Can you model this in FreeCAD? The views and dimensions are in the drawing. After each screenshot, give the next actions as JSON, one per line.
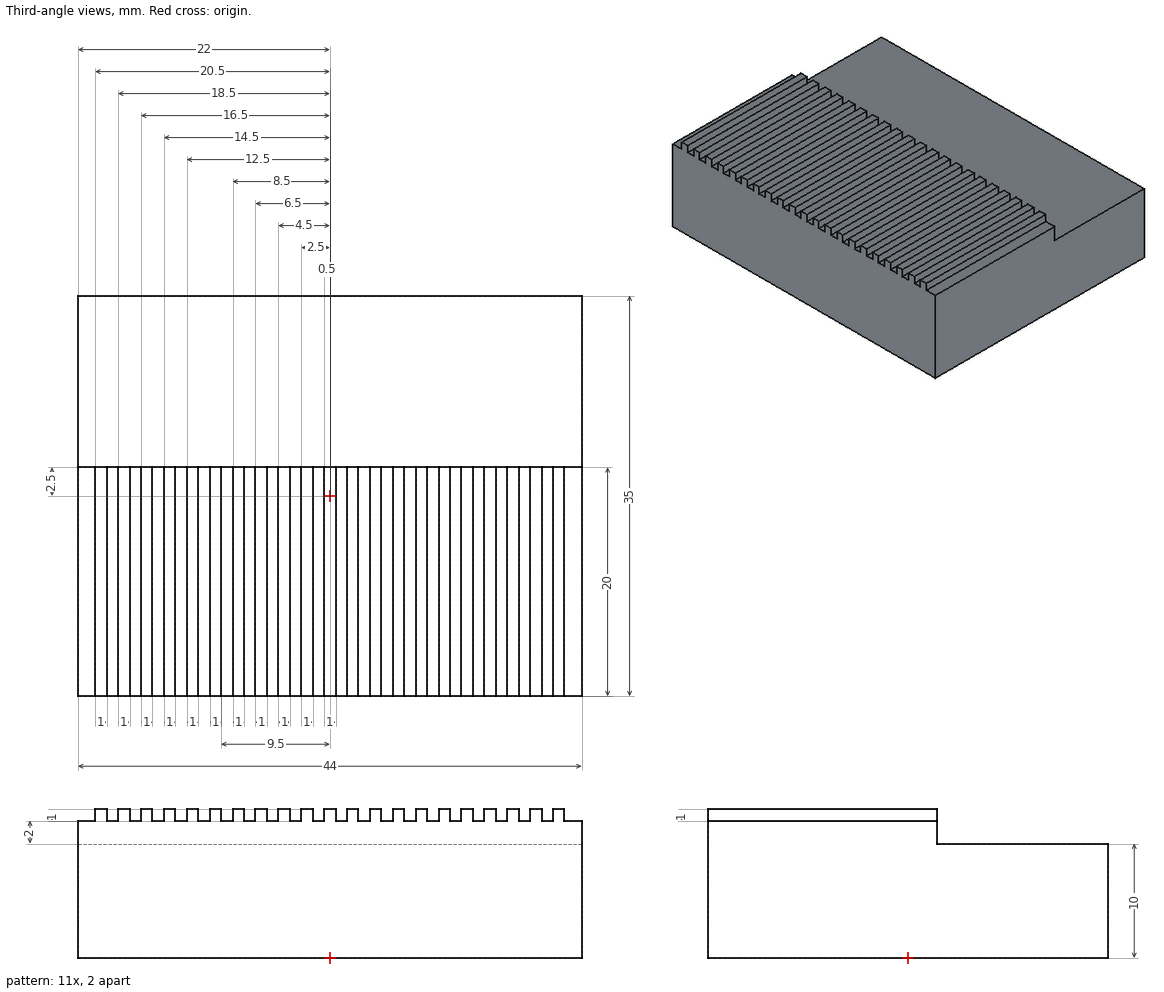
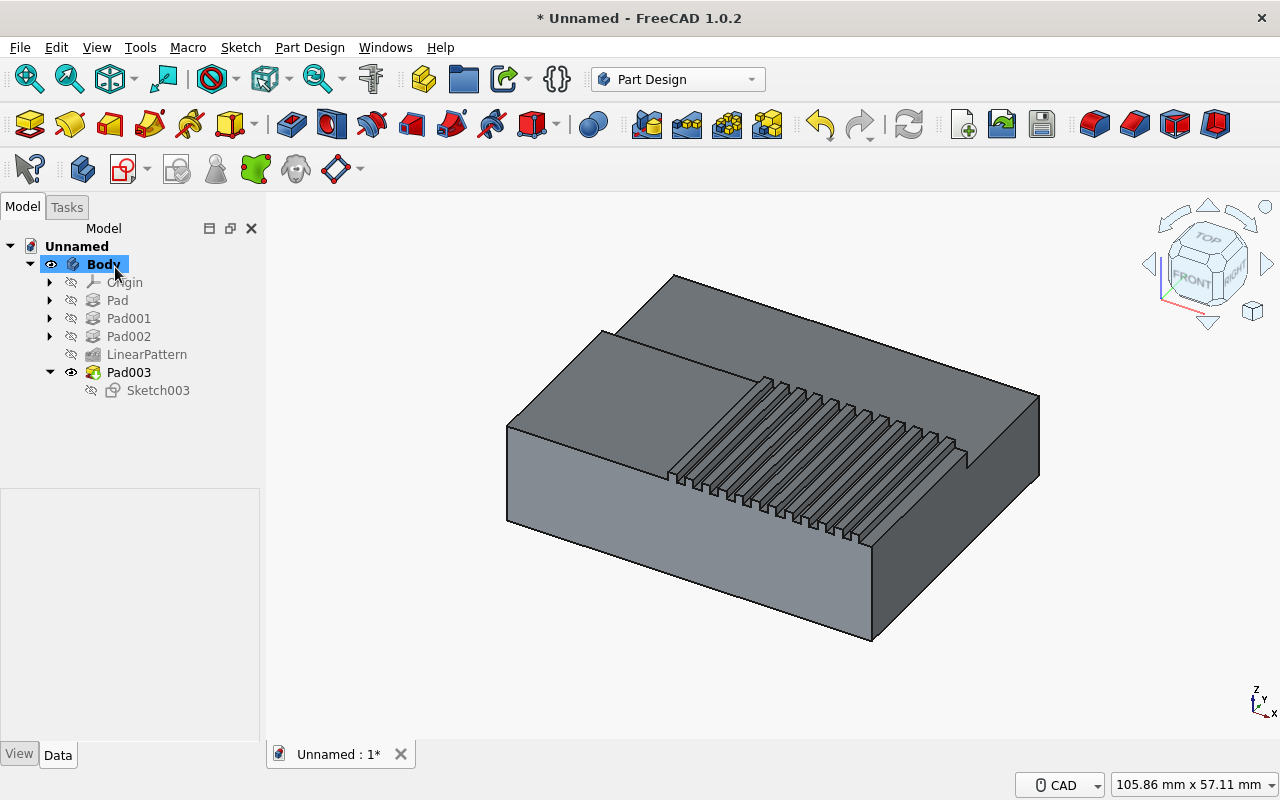
{"action": "left_click", "coordinate": [635, 404]}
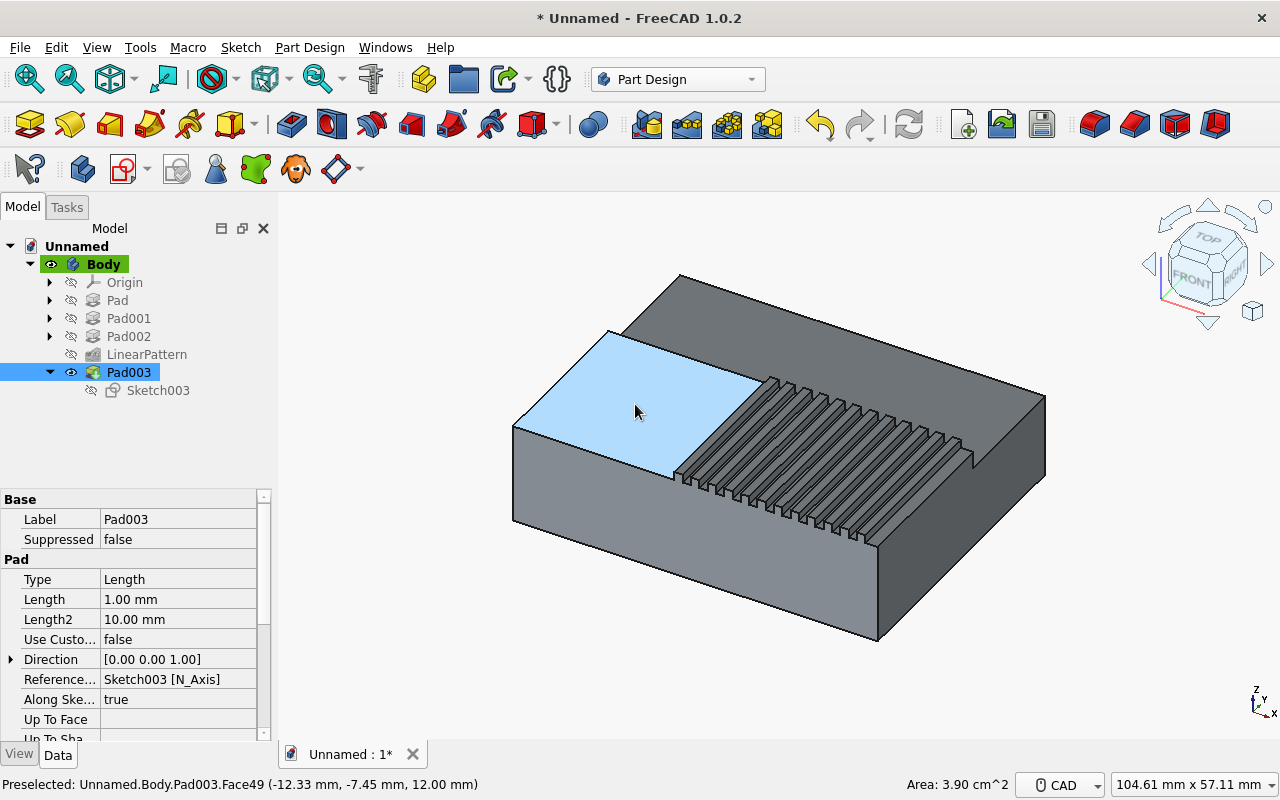
{"action": "left_click", "coordinate": [124, 170]}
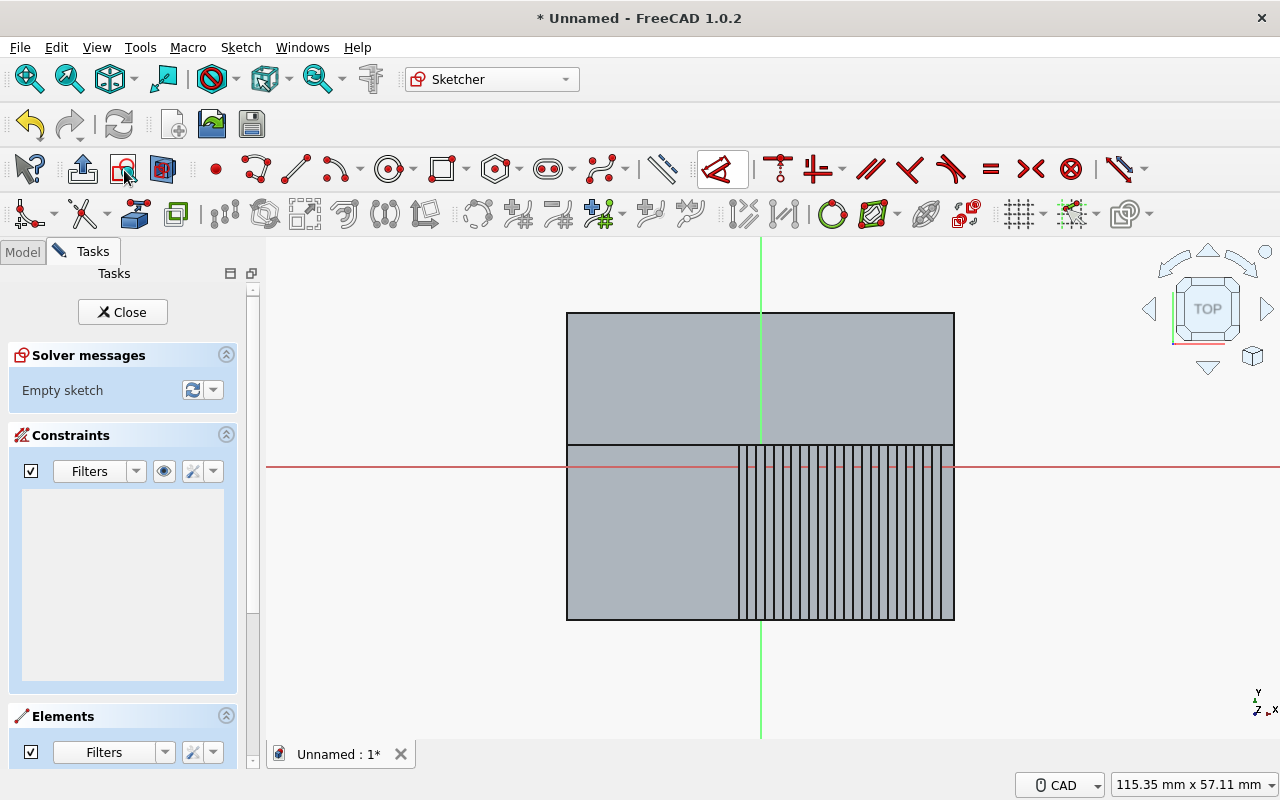
{"action": "left_click", "coordinate": [164, 170]}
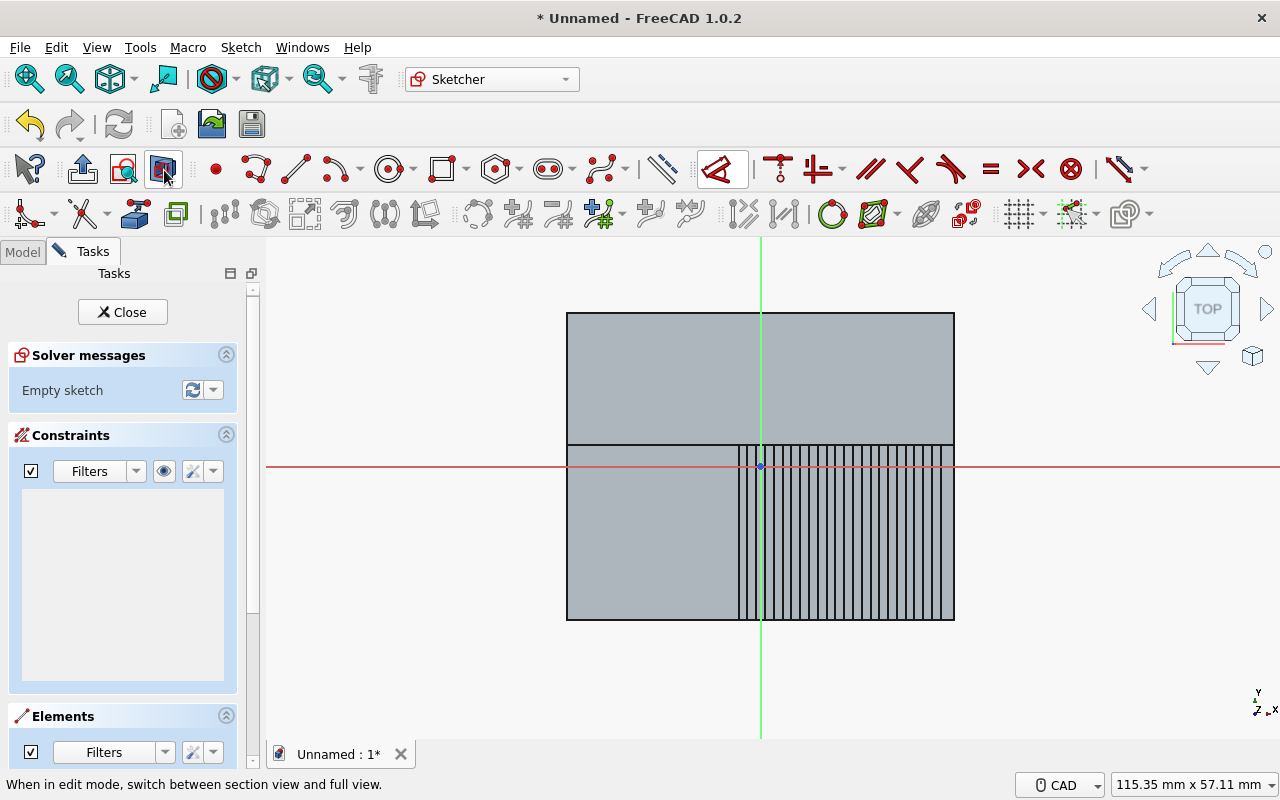
{"action": "scroll", "coordinate": [785, 587], "scroll_direction": "up", "scroll_amount": 3}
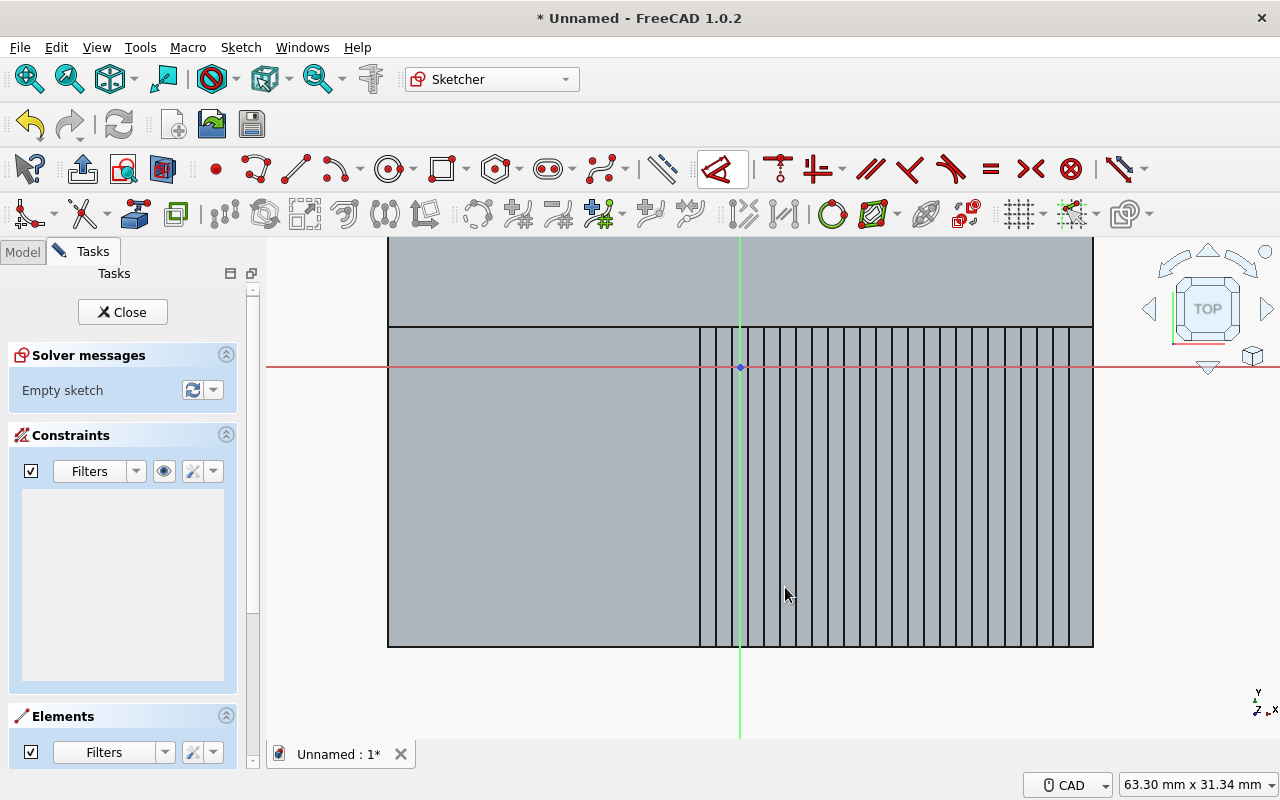
{"action": "left_click", "coordinate": [442, 170]}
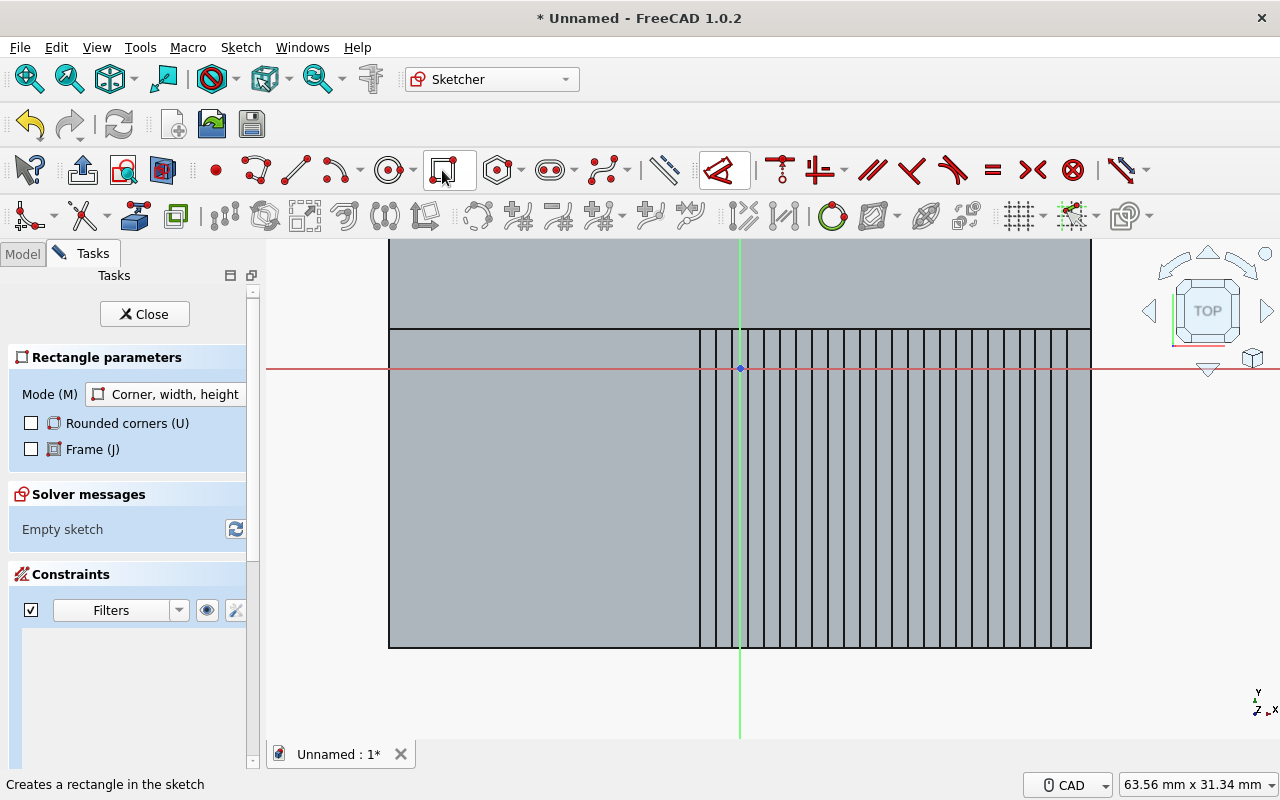
{"action": "left_click", "coordinate": [669, 329]}
{"action": "mouse_move", "coordinate": [685, 648]}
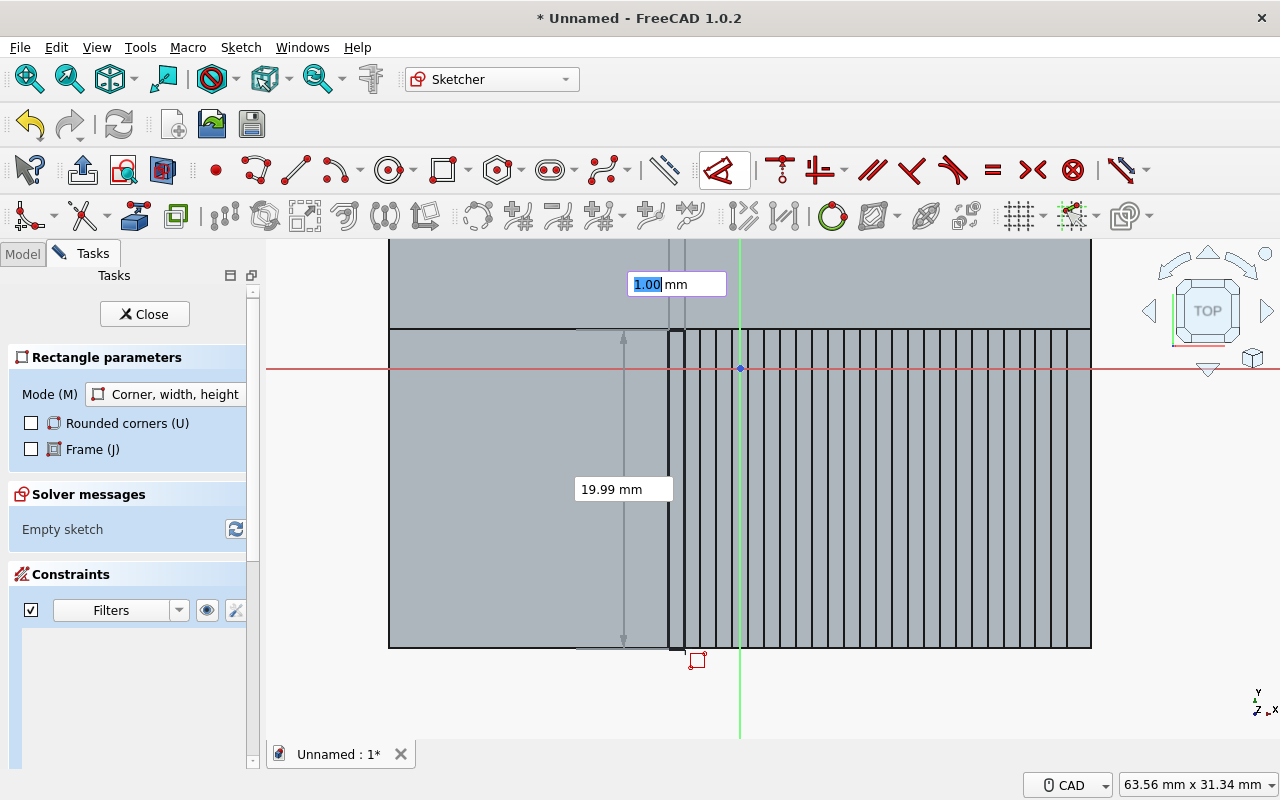
{"action": "type", "text": "1"}
{"action": "key", "text": "Tab"}
{"action": "type", "text": "20"}
{"action": "key", "text": "Return"}
{"action": "key", "text": "Escape"}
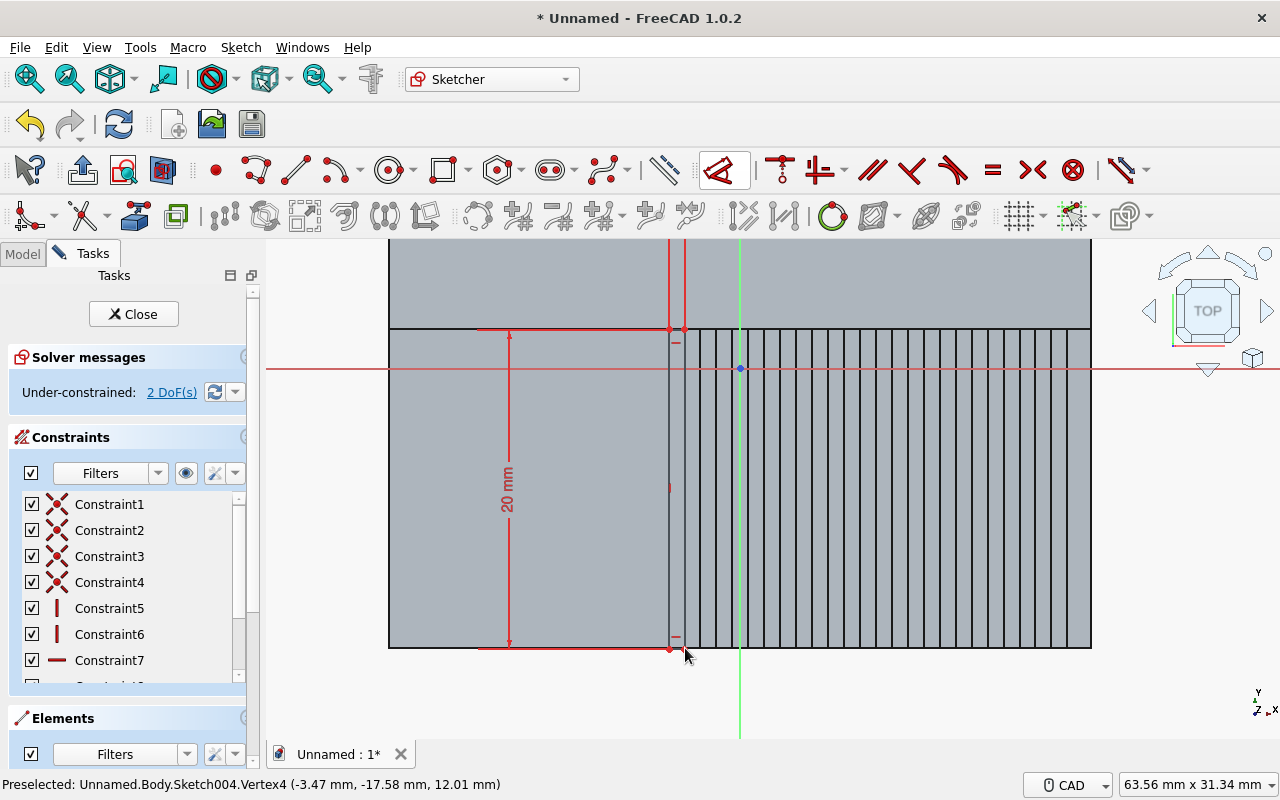
{"action": "left_click", "coordinate": [669, 330]}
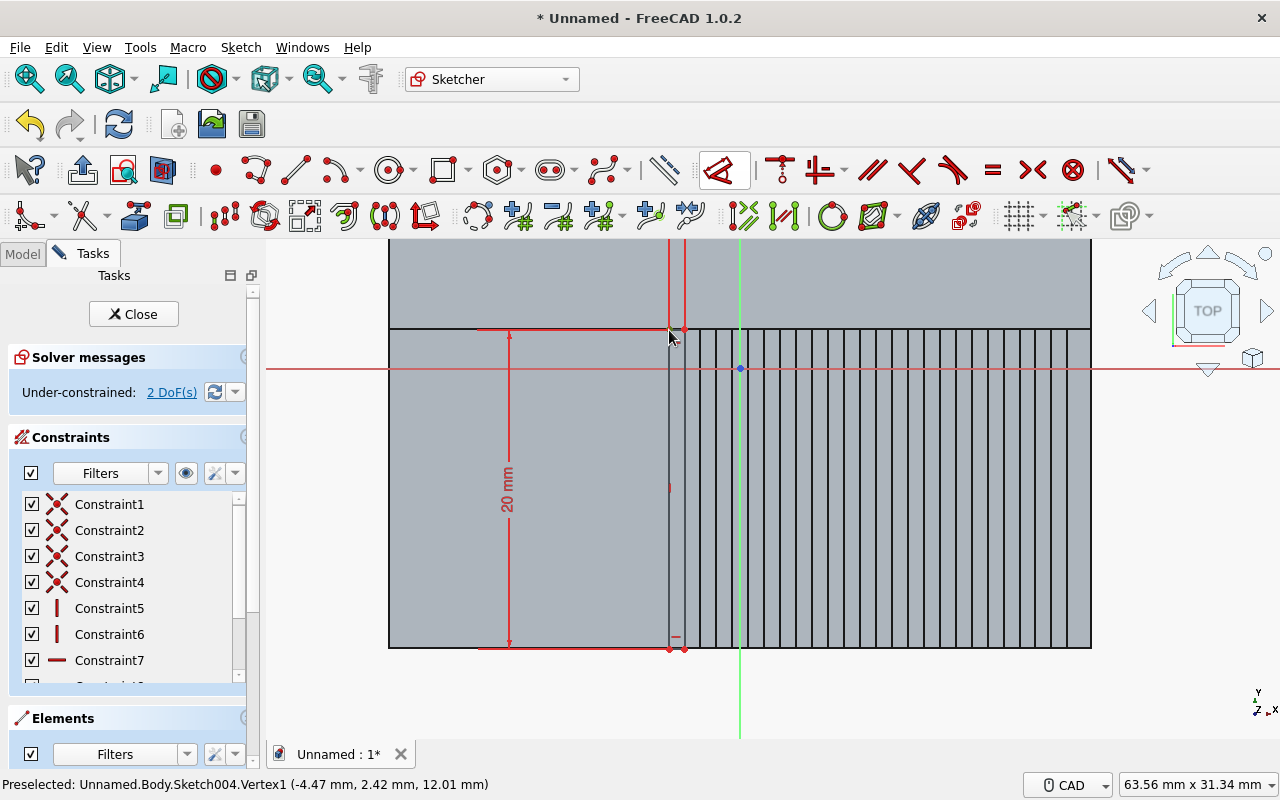
{"action": "key", "text": "l"}